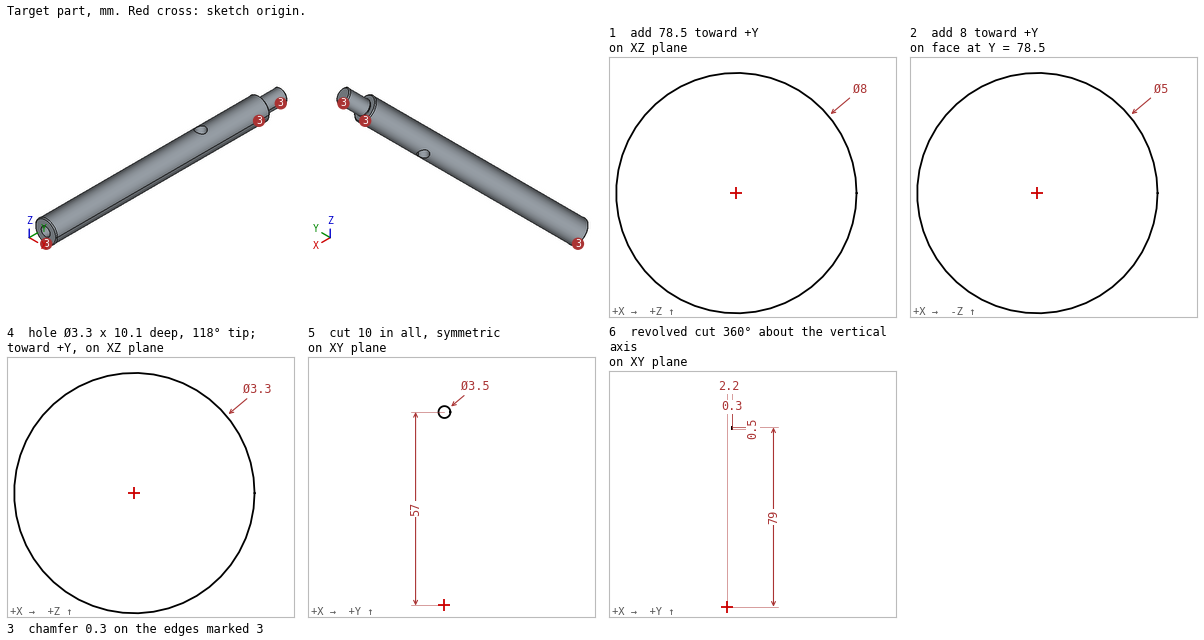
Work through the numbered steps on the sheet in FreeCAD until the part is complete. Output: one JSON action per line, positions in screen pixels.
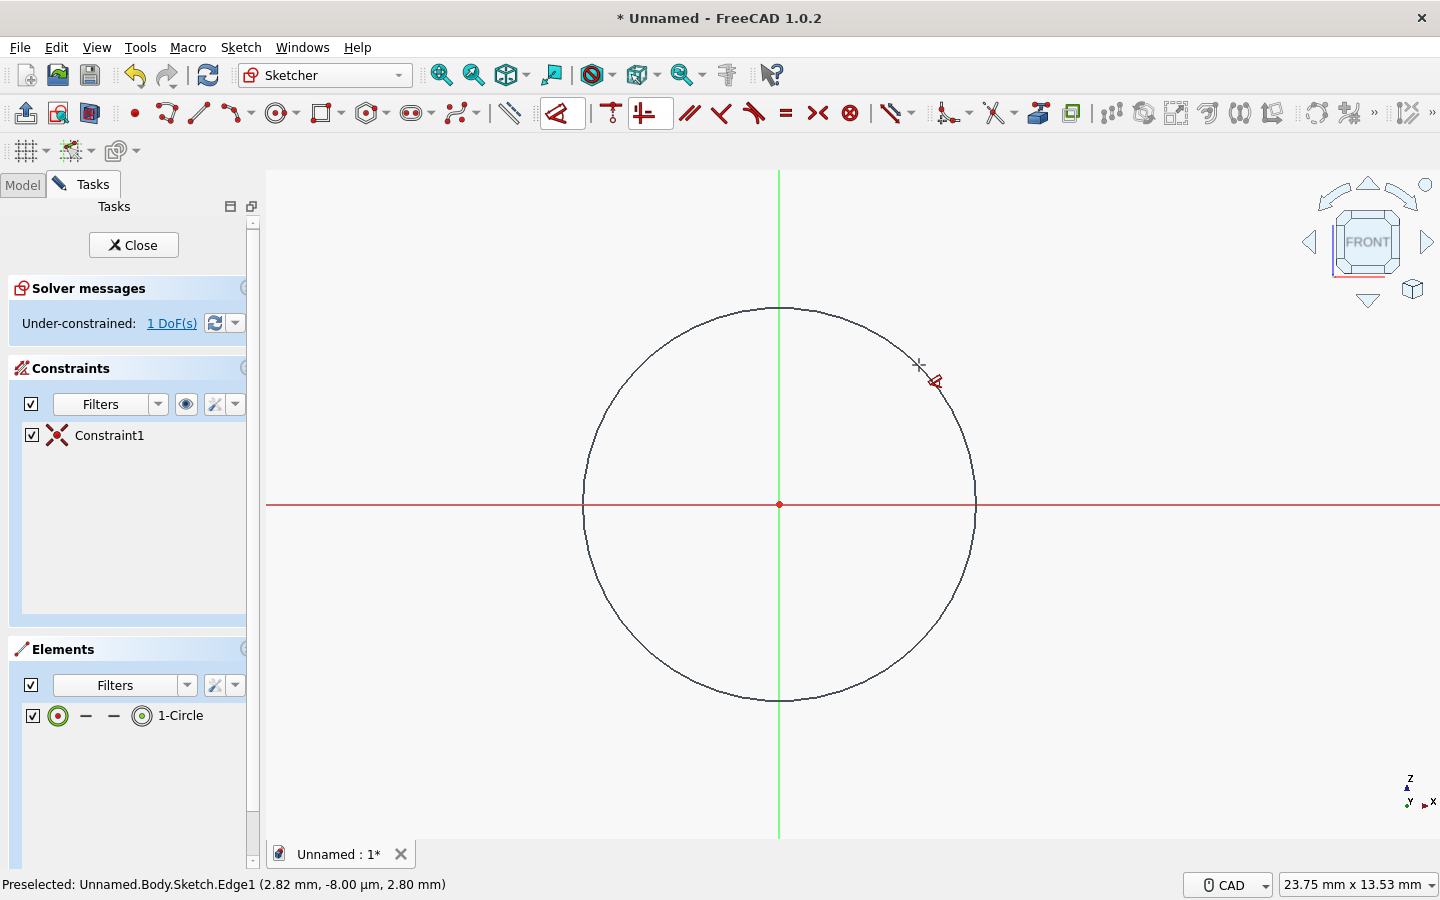
{"action": "left_click", "coordinate": [918, 365]}
{"action": "left_click", "coordinate": [941, 342]}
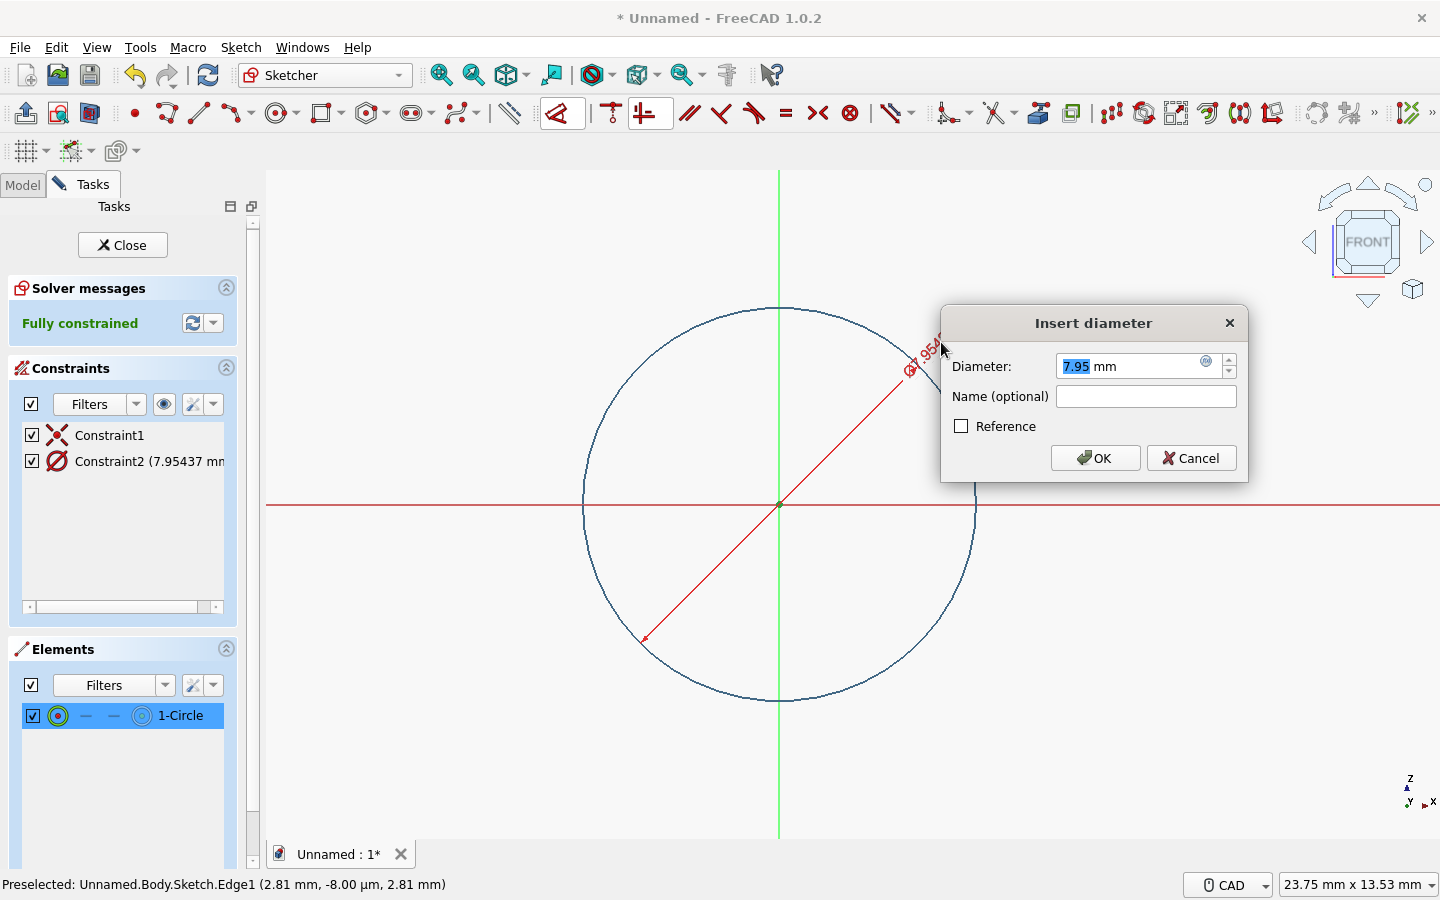
{"action": "type", "text": "8"}
{"action": "key", "text": "Return"}
{"action": "key", "text": "Escape"}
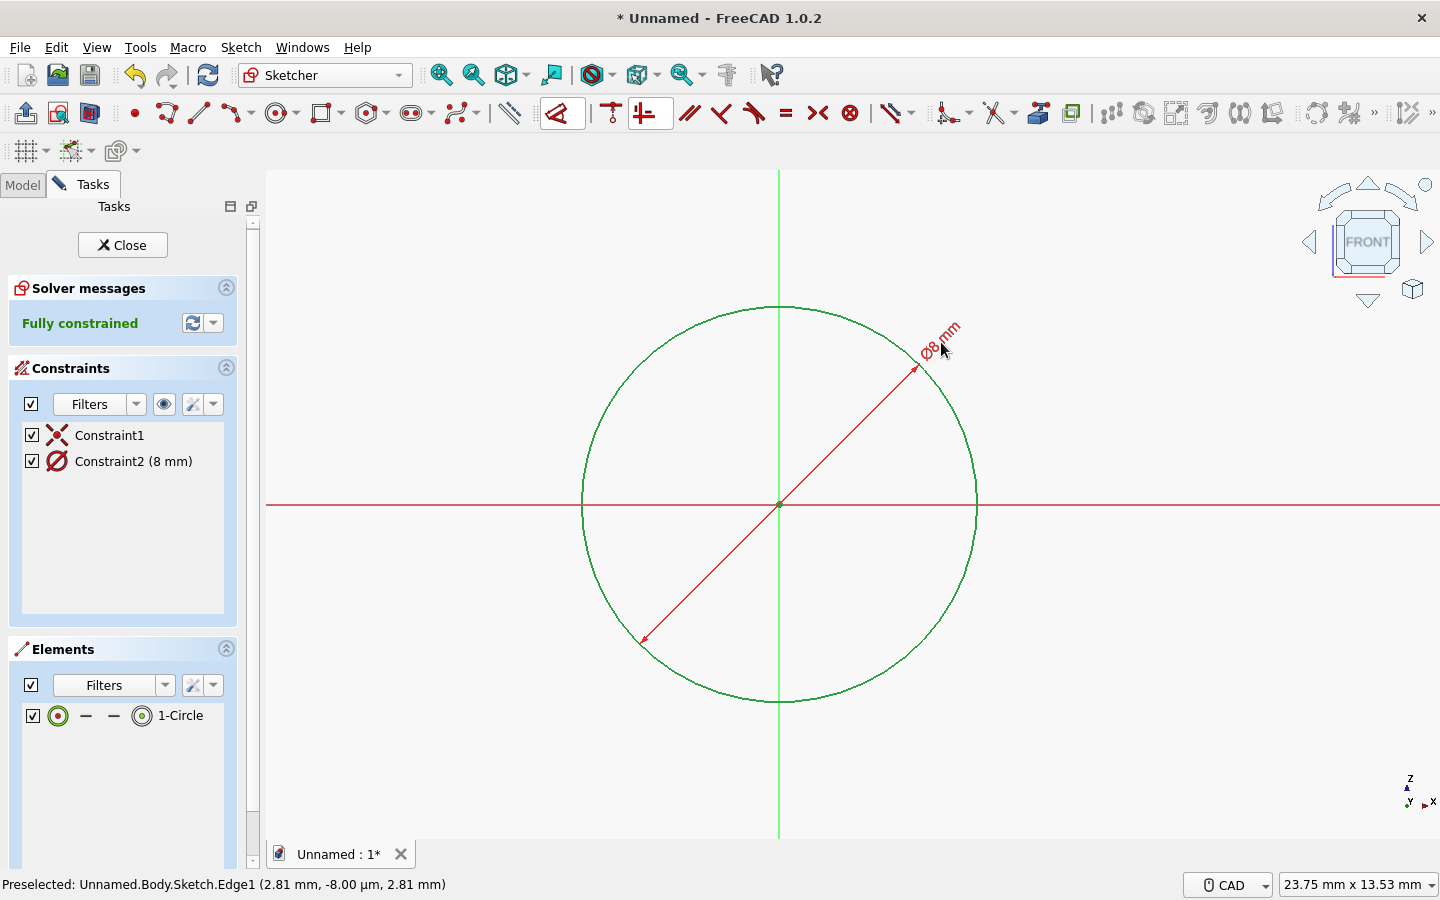
{"action": "left_click", "coordinate": [123, 245]}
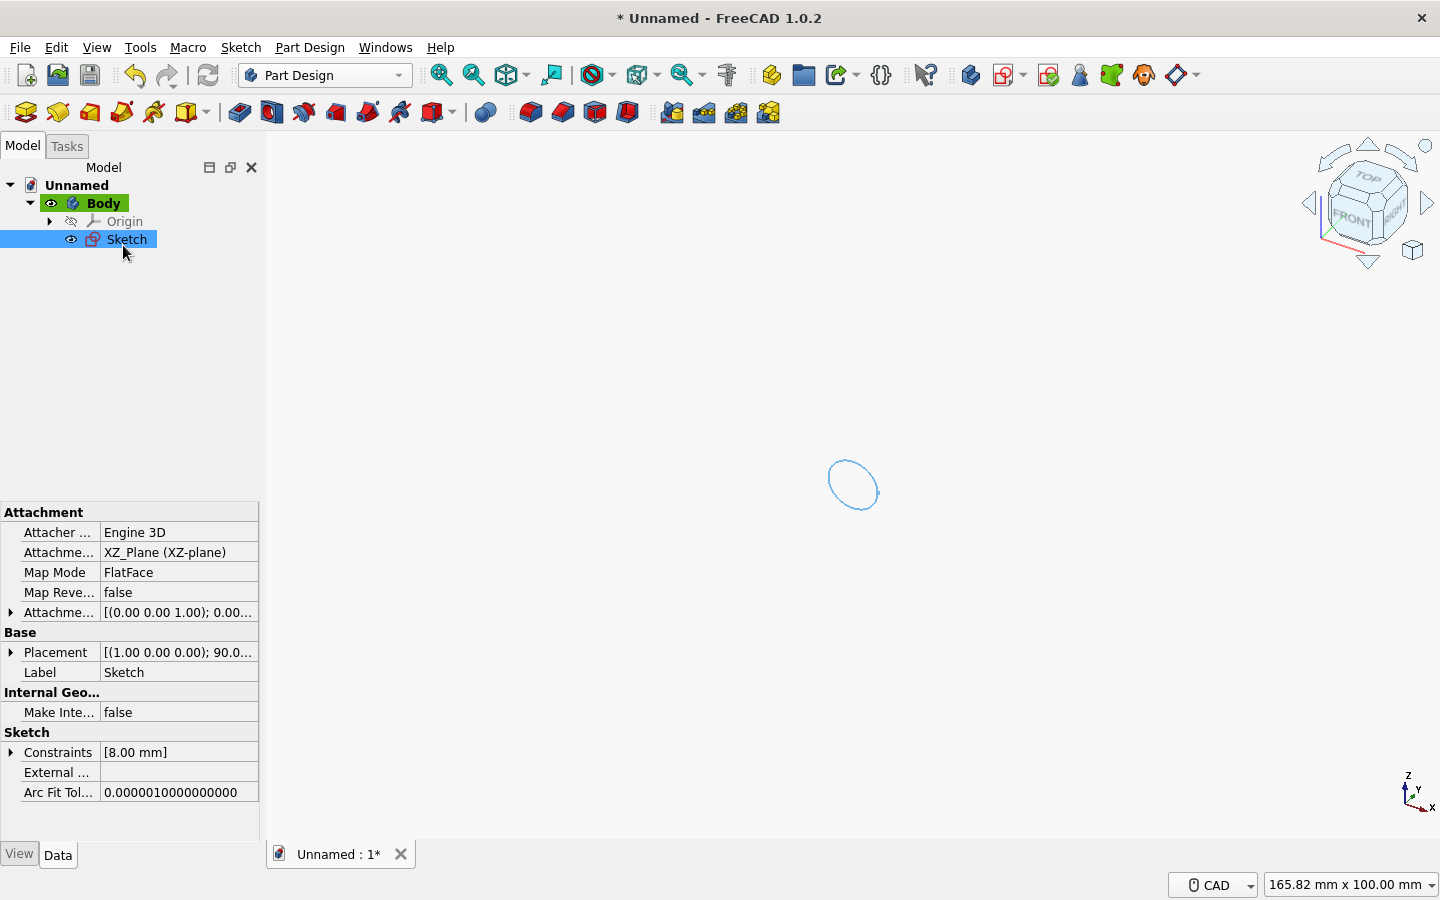
{"action": "left_click", "coordinate": [26, 112]}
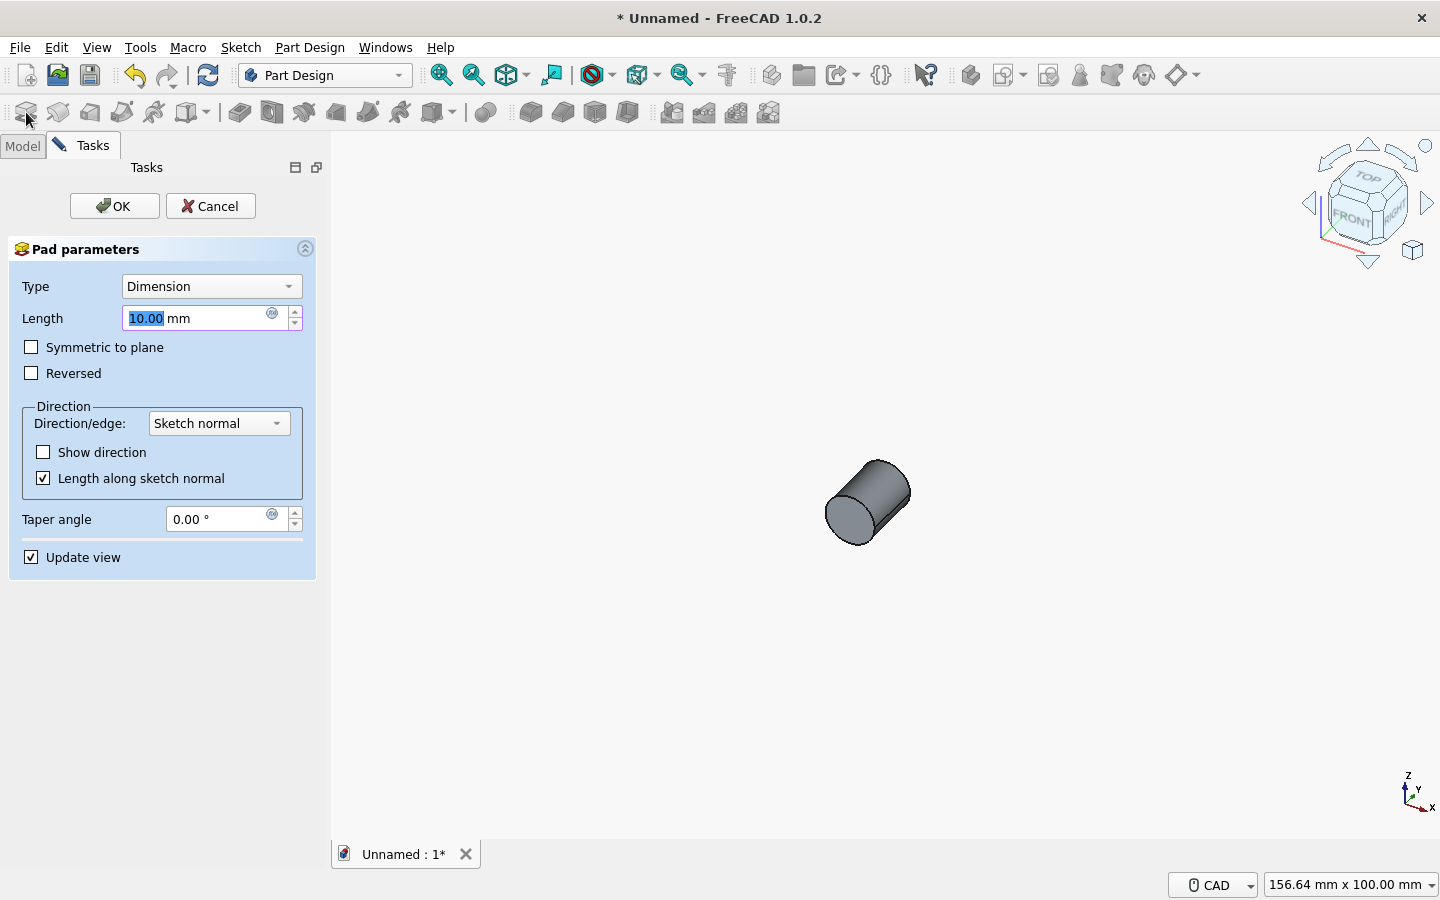
{"action": "type", "text": "78.5"}
{"action": "key", "text": "Tab"}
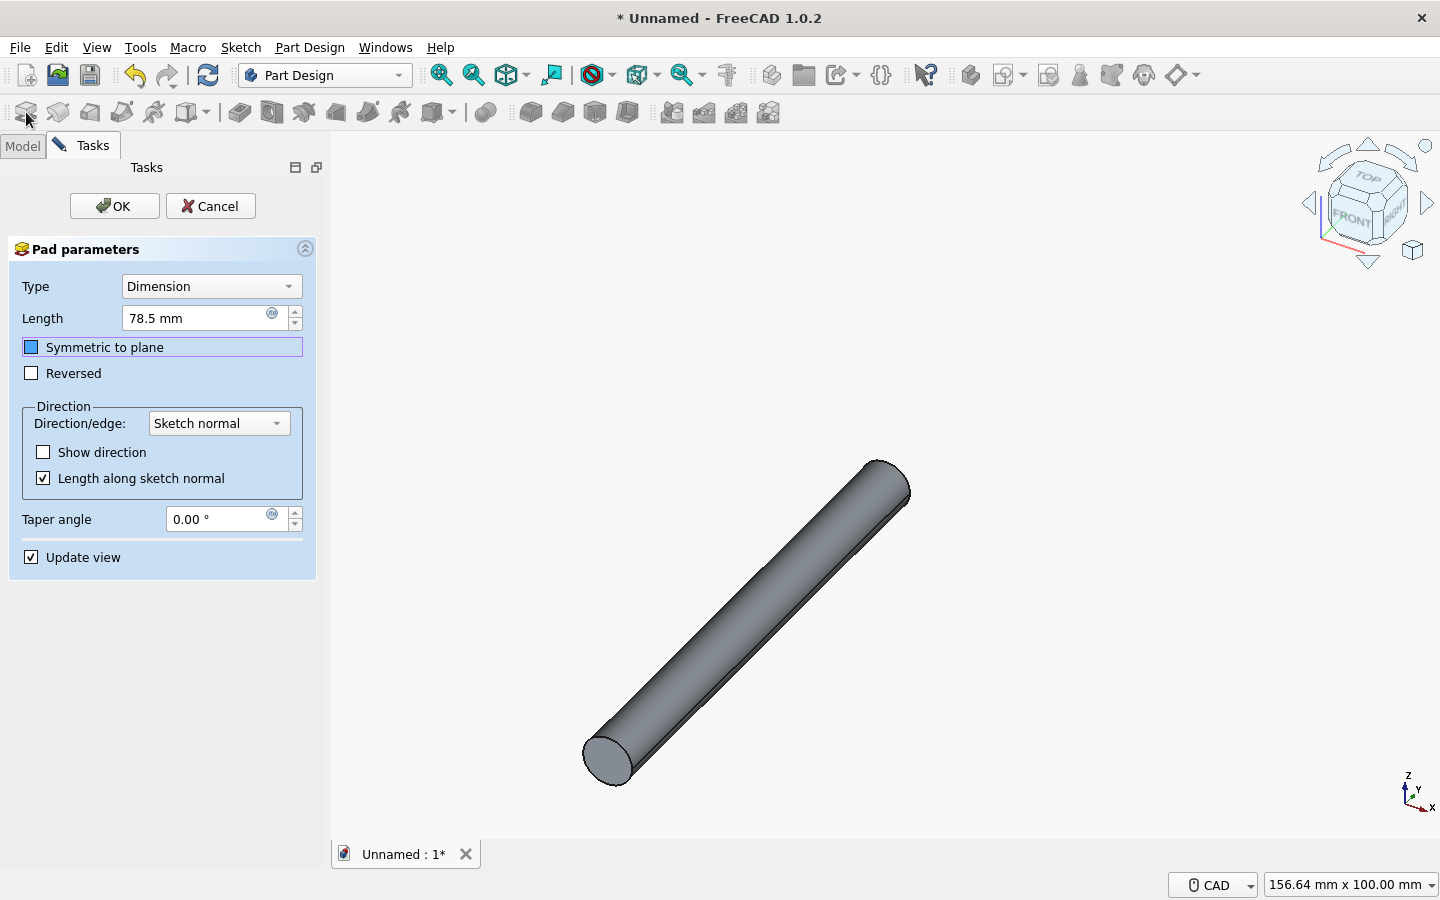
{"action": "left_click", "coordinate": [30, 373]}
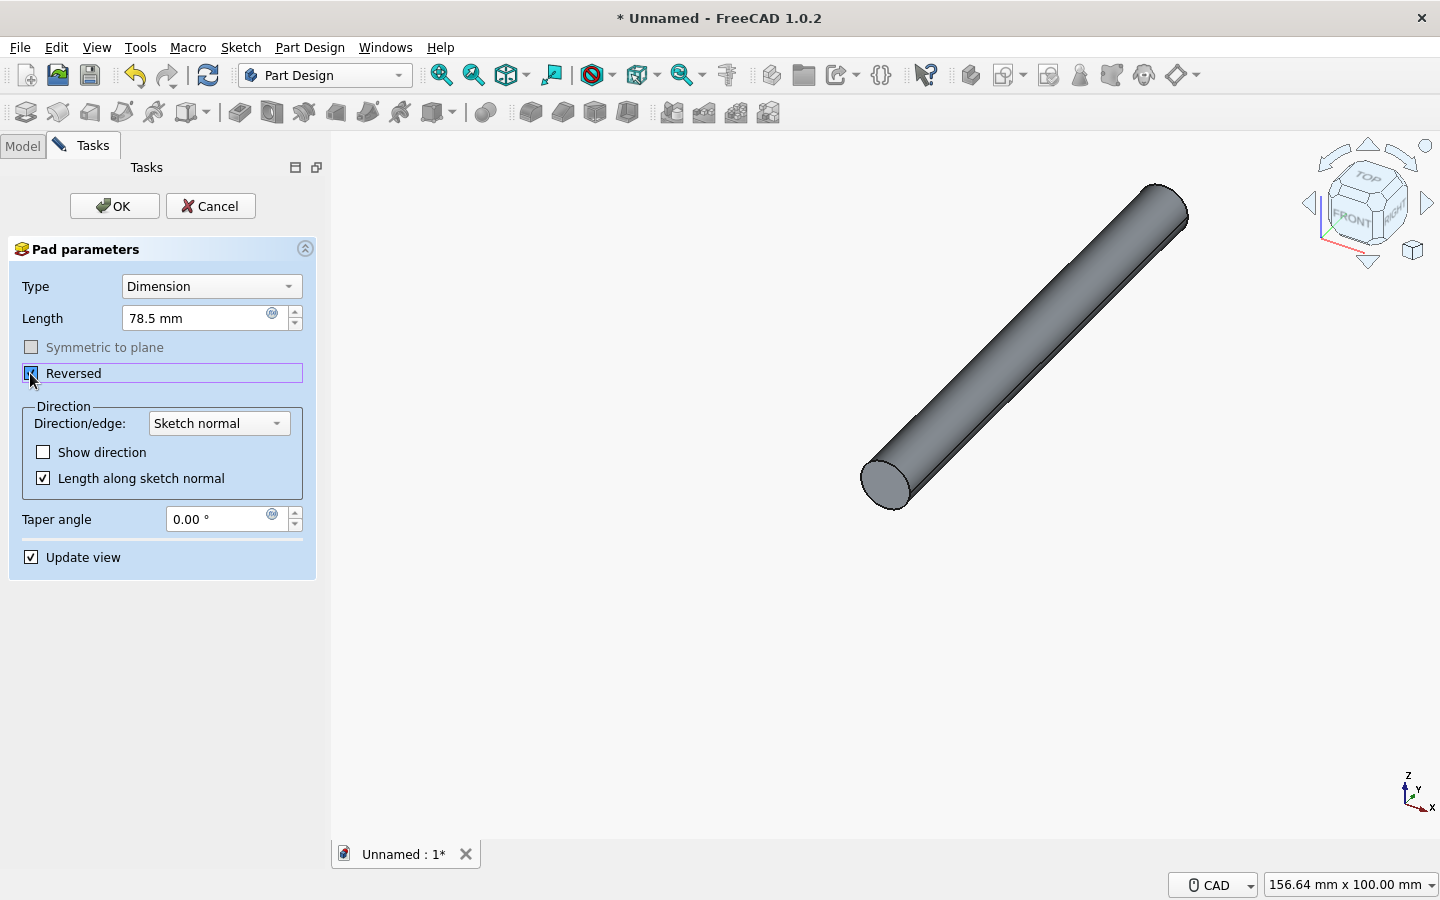
{"action": "left_click", "coordinate": [115, 206]}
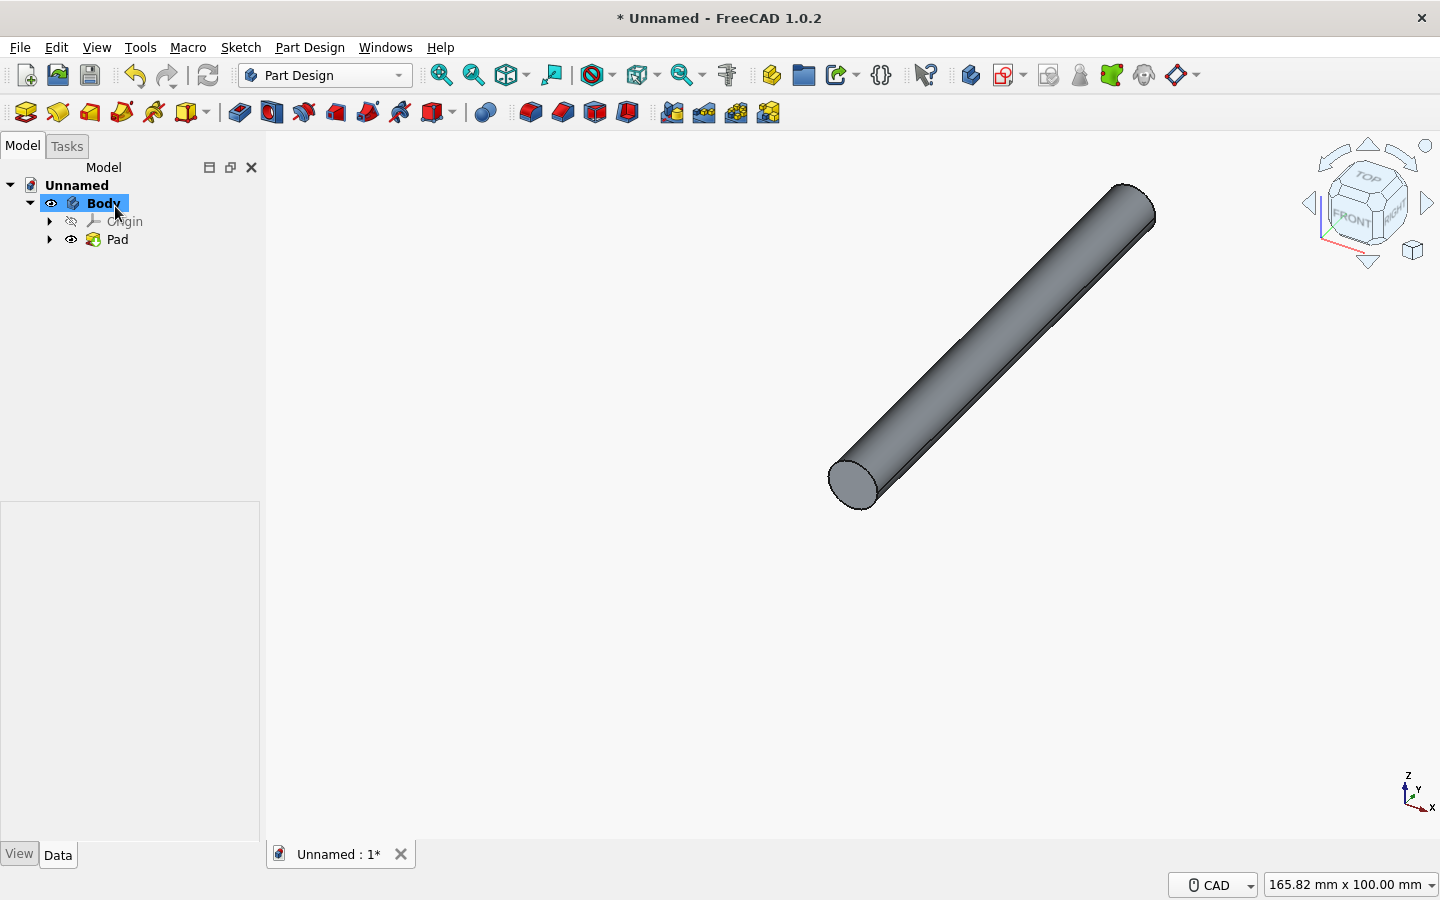
{"action": "key", "text": "4"}